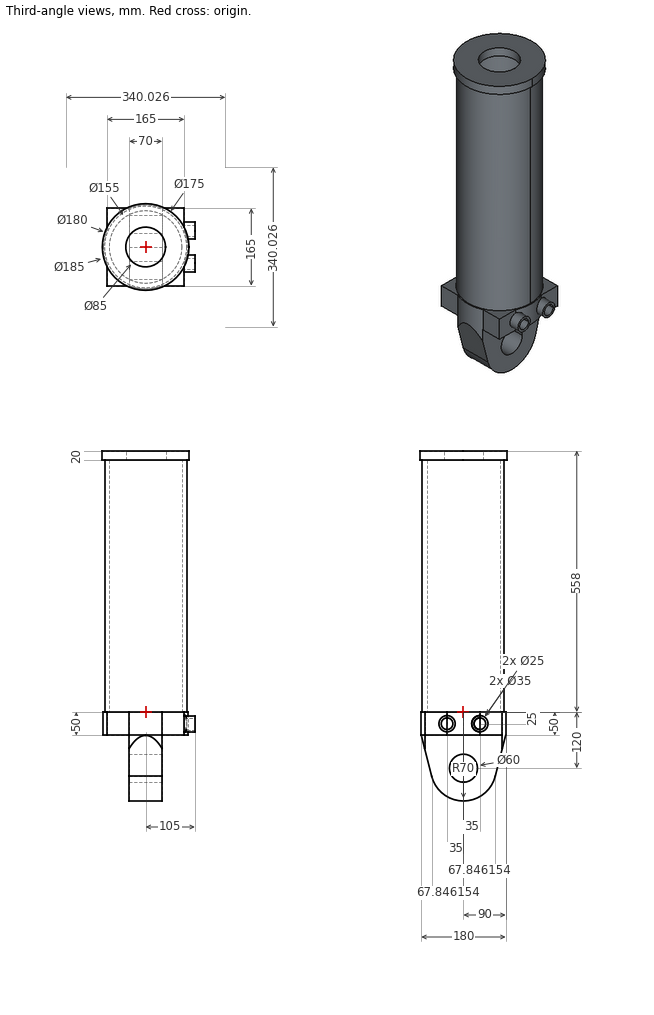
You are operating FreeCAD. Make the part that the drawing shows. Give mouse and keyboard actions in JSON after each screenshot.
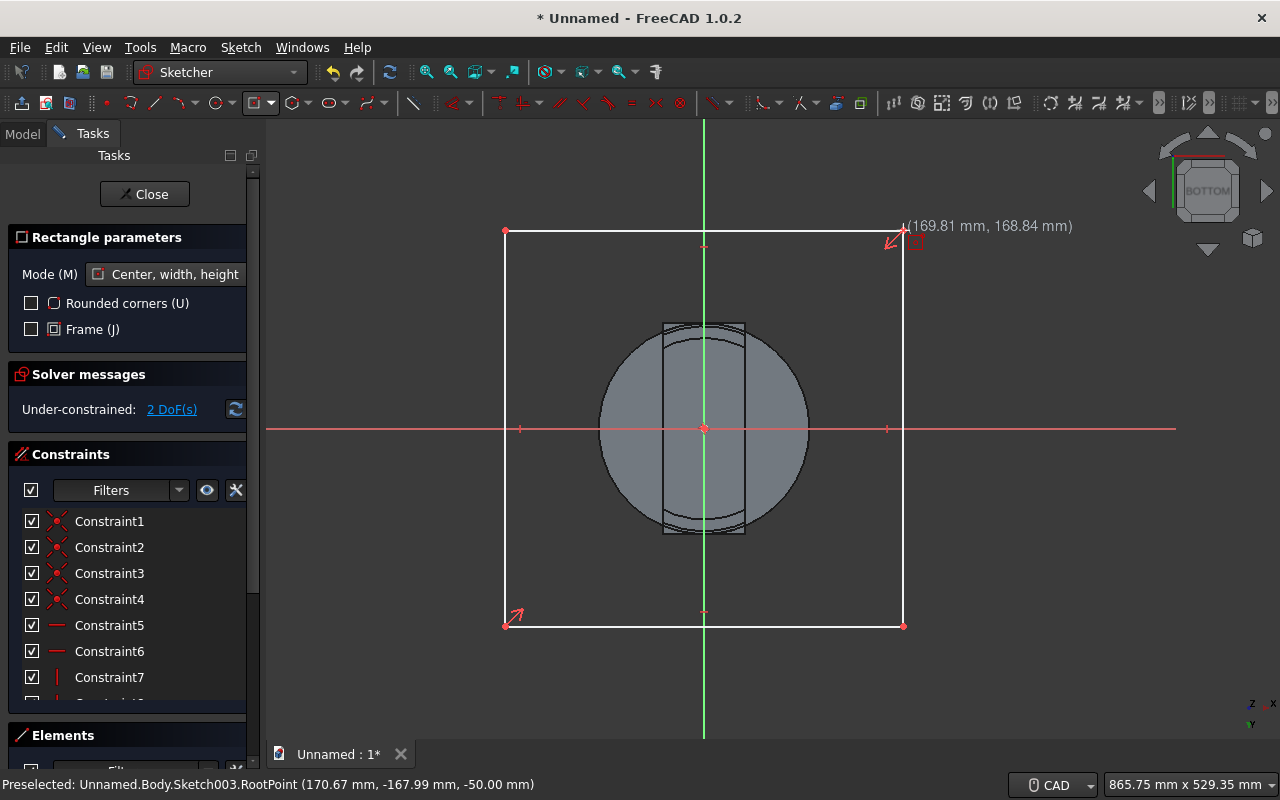
{"action": "left_click", "coordinate": [216, 104]}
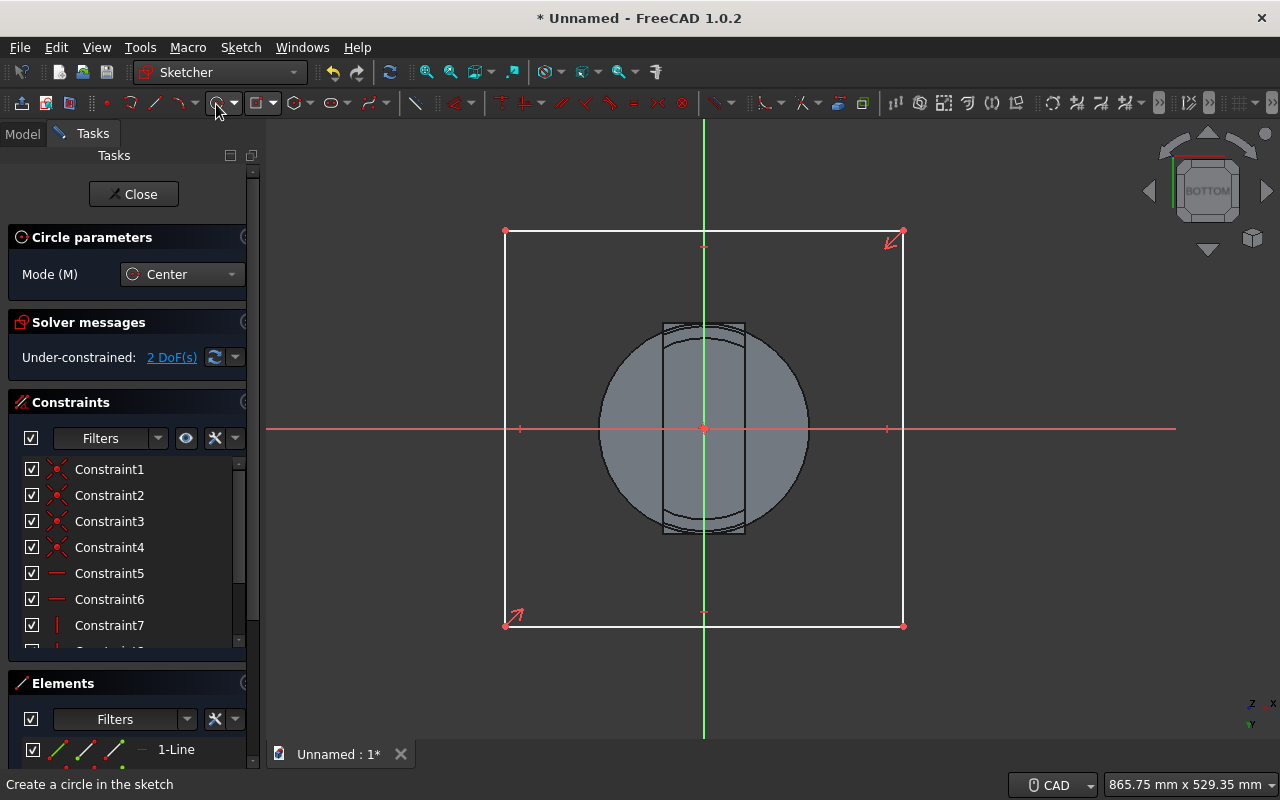
{"action": "left_click", "coordinate": [704, 429]}
{"action": "left_click", "coordinate": [779, 354]}
{"action": "key", "text": "Escape"}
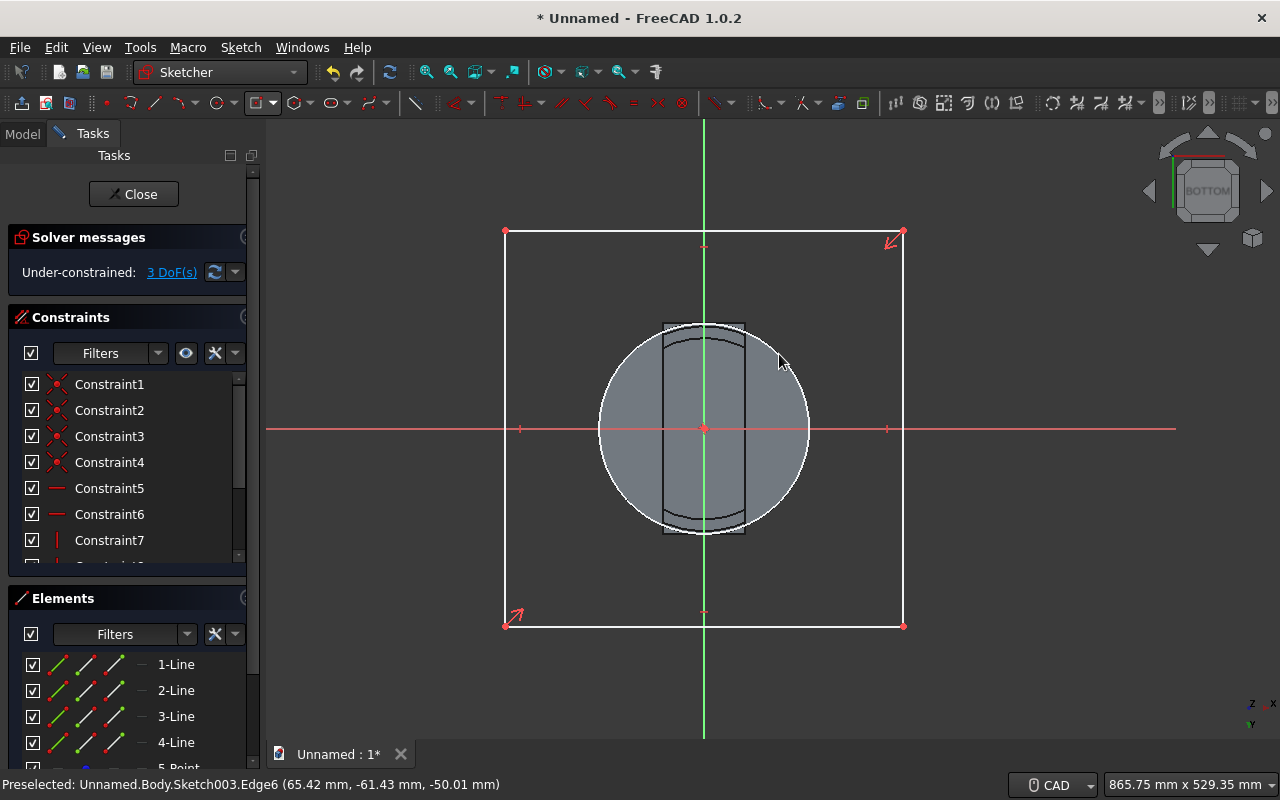
{"action": "left_click", "coordinate": [454, 104]}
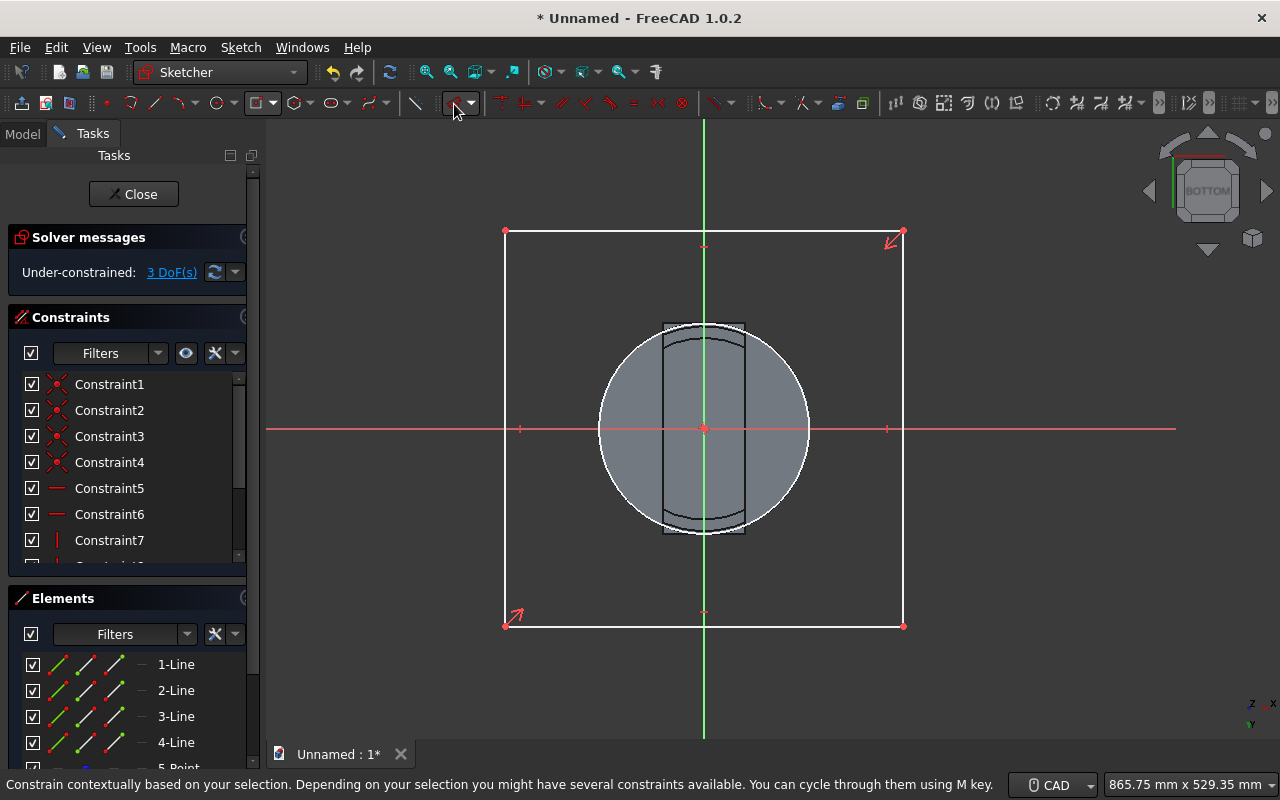
{"action": "left_click", "coordinate": [778, 354]}
{"action": "left_click", "coordinate": [800, 331]}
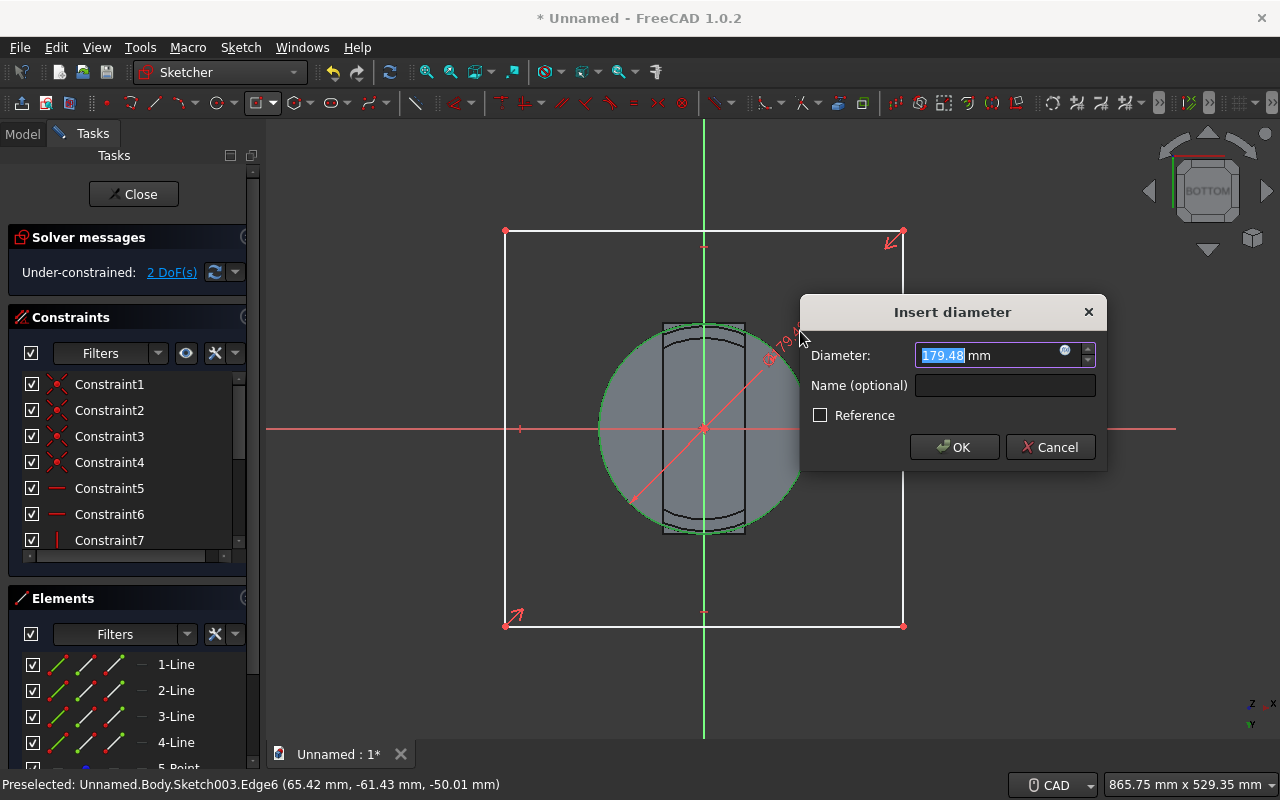
{"action": "type", "text": "180"}
{"action": "key", "text": "Return"}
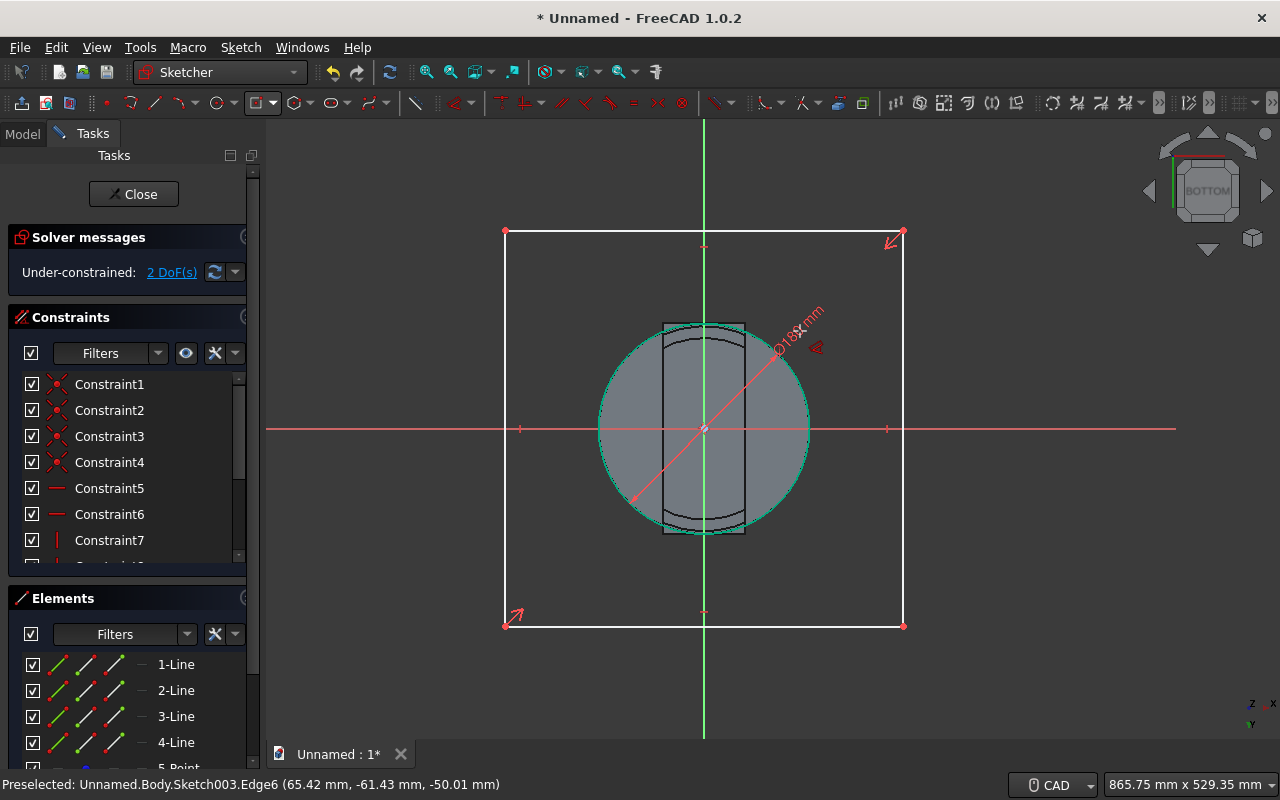
{"action": "left_click", "coordinate": [625, 627]}
{"action": "left_click", "coordinate": [613, 661]}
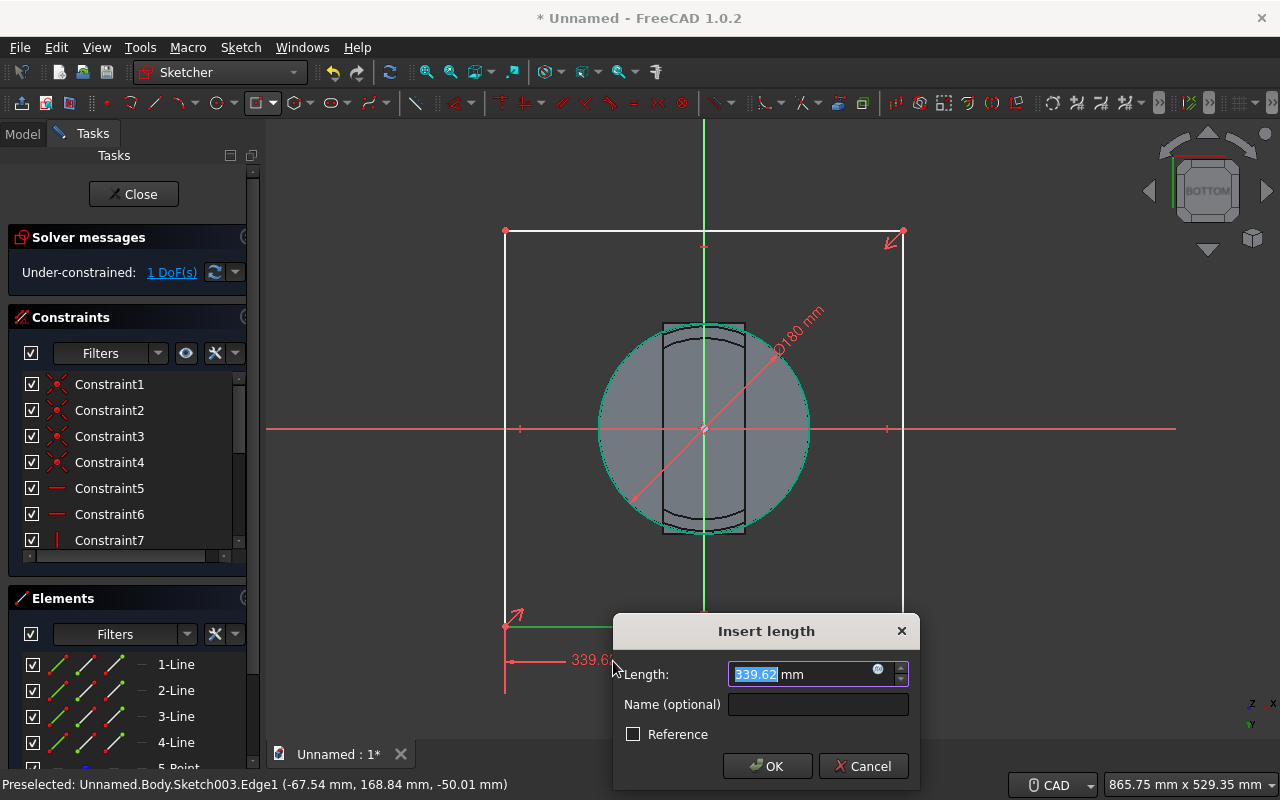
{"action": "type", "text": "340.026"}
{"action": "key", "text": "Return"}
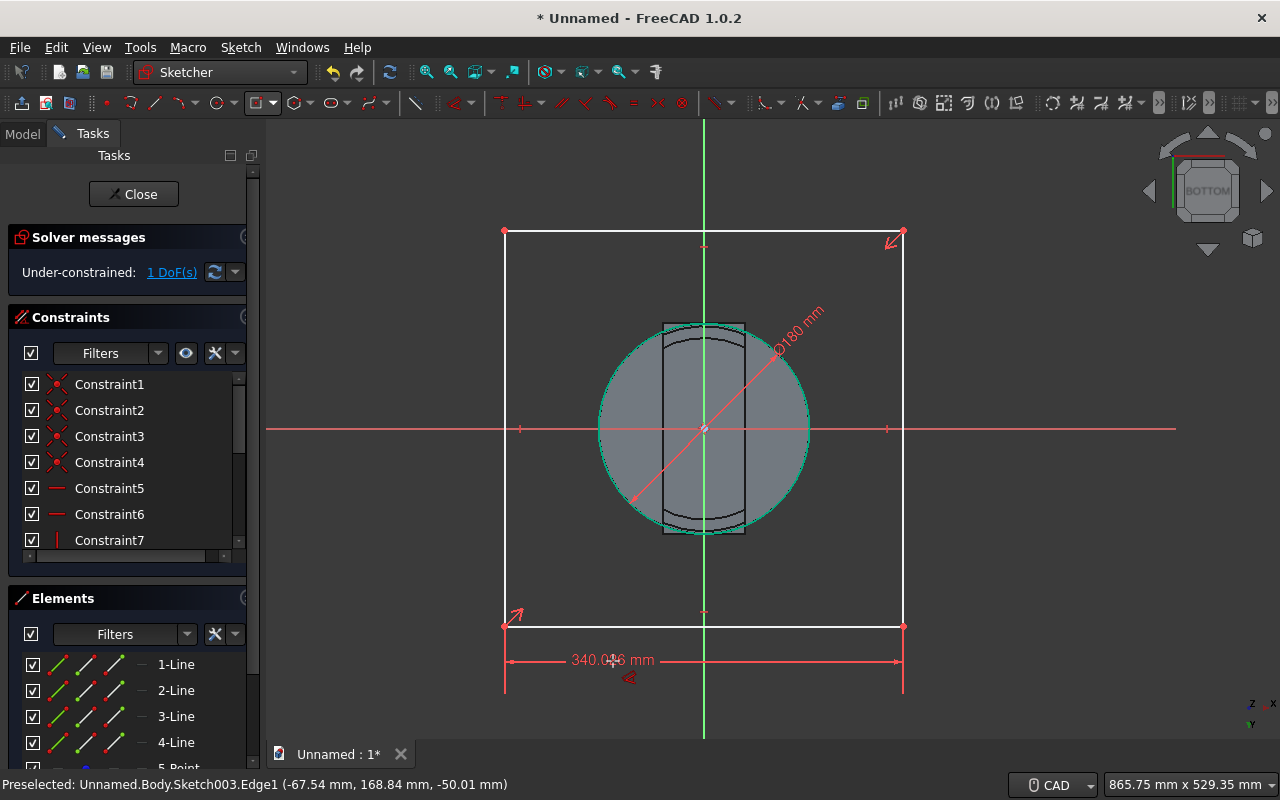
{"action": "left_click", "coordinate": [903, 508]}
{"action": "left_click", "coordinate": [937, 338]}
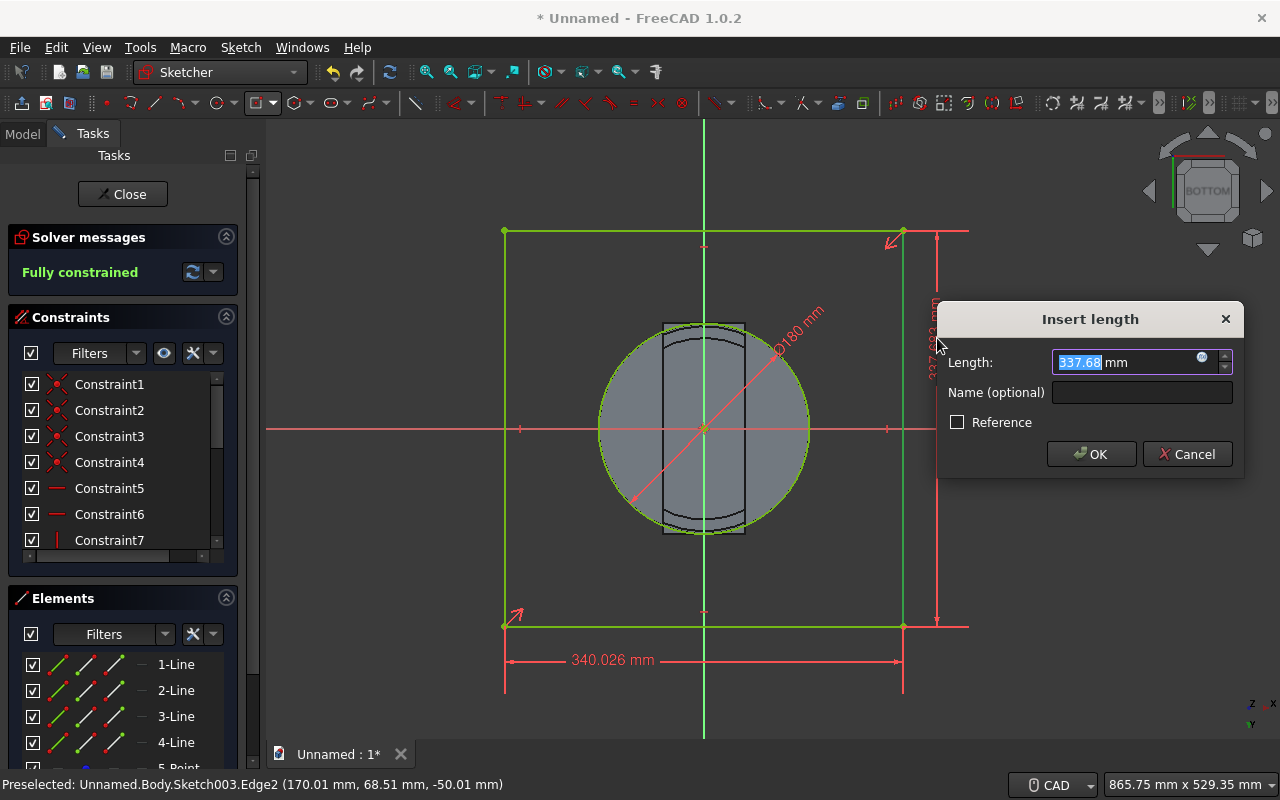
{"action": "type", "text": "340.026"}
{"action": "key", "text": "Return"}
{"action": "key", "text": "Escape"}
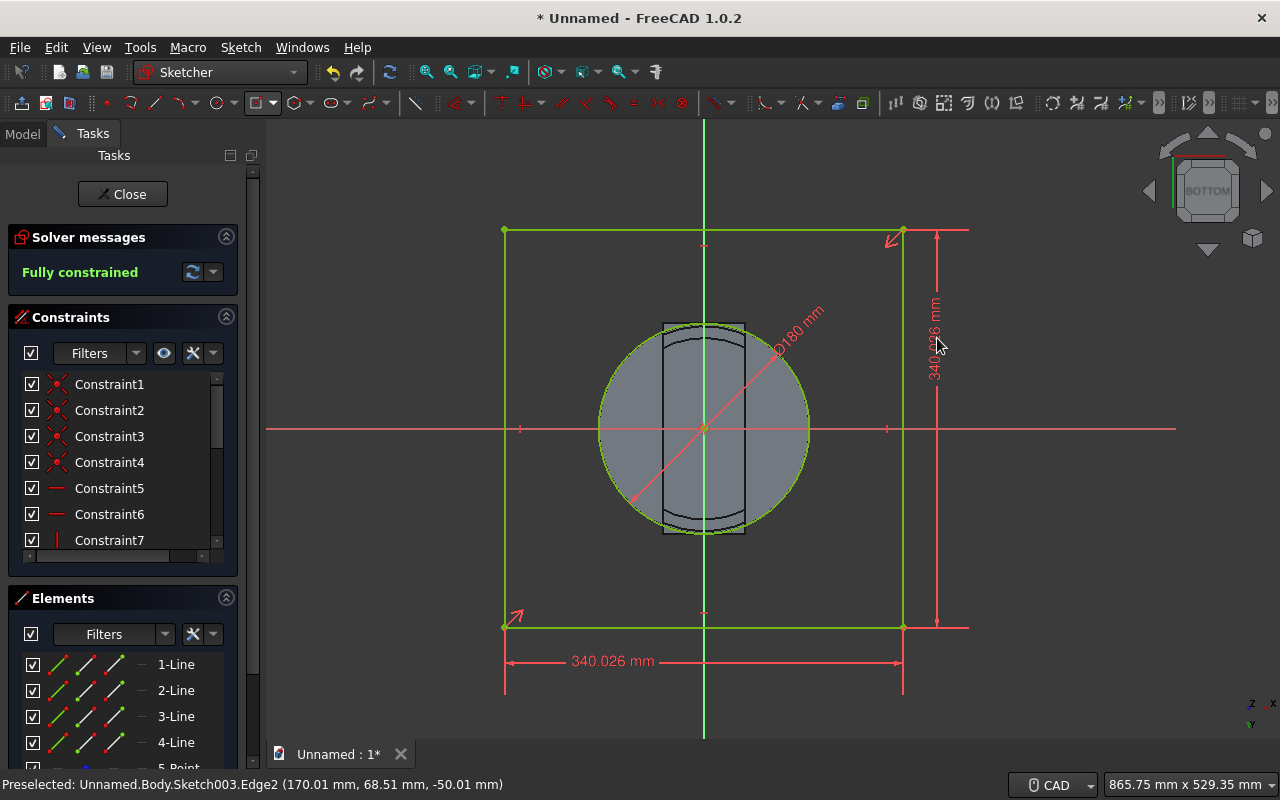
{"action": "left_click", "coordinate": [123, 194]}